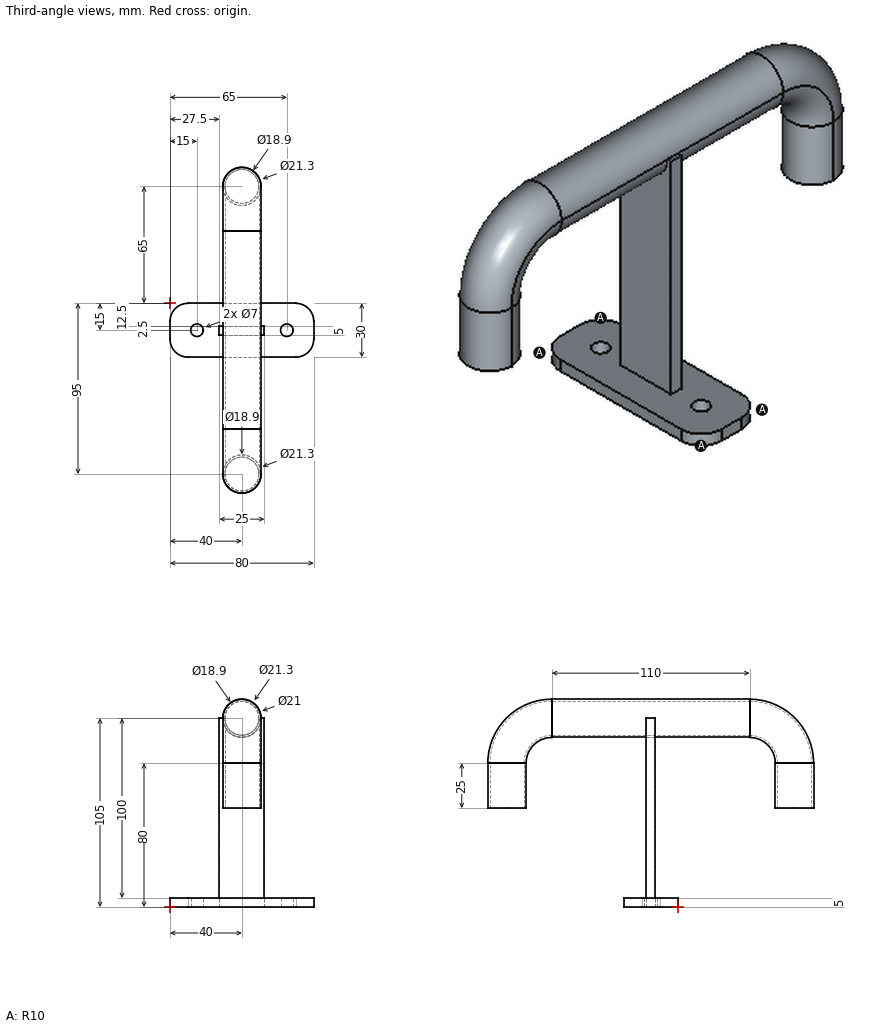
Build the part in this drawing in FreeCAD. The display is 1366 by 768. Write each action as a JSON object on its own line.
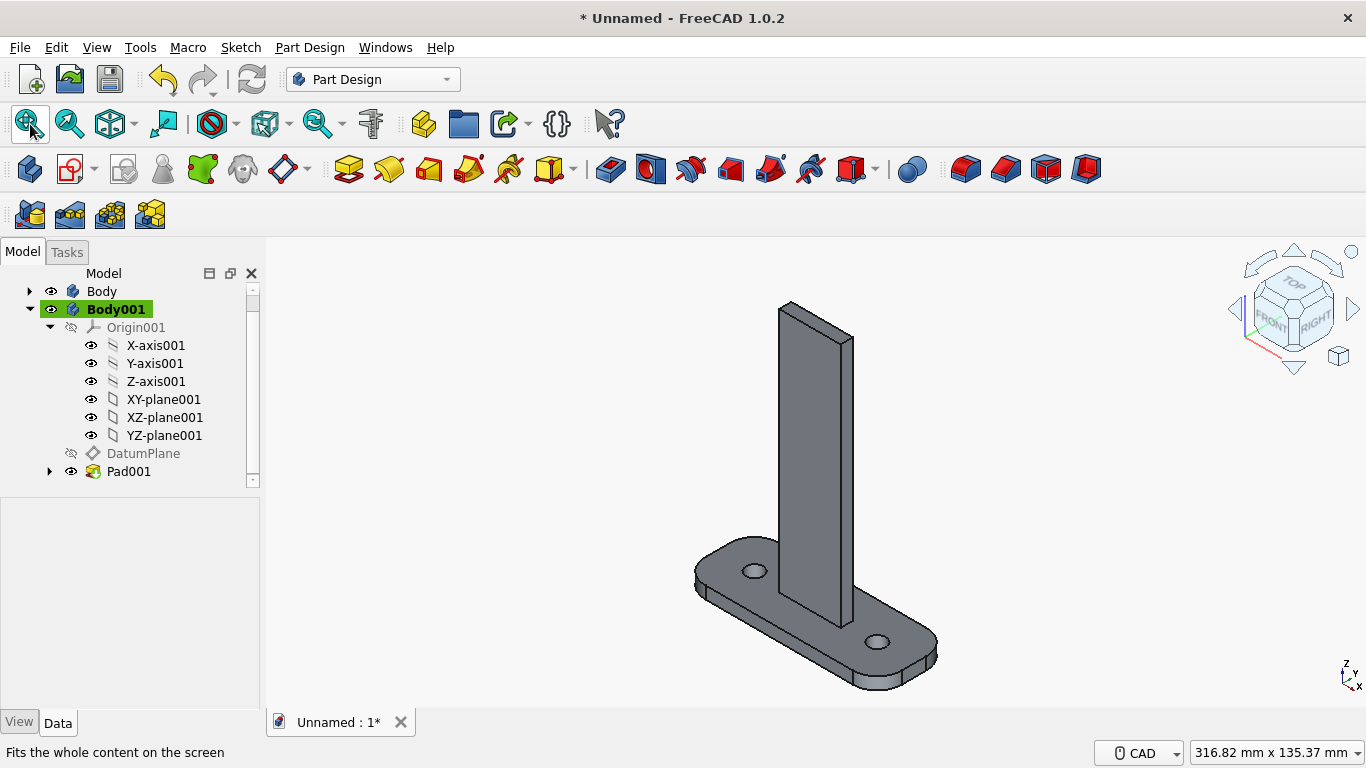
{"action": "left_click", "coordinate": [810, 386]}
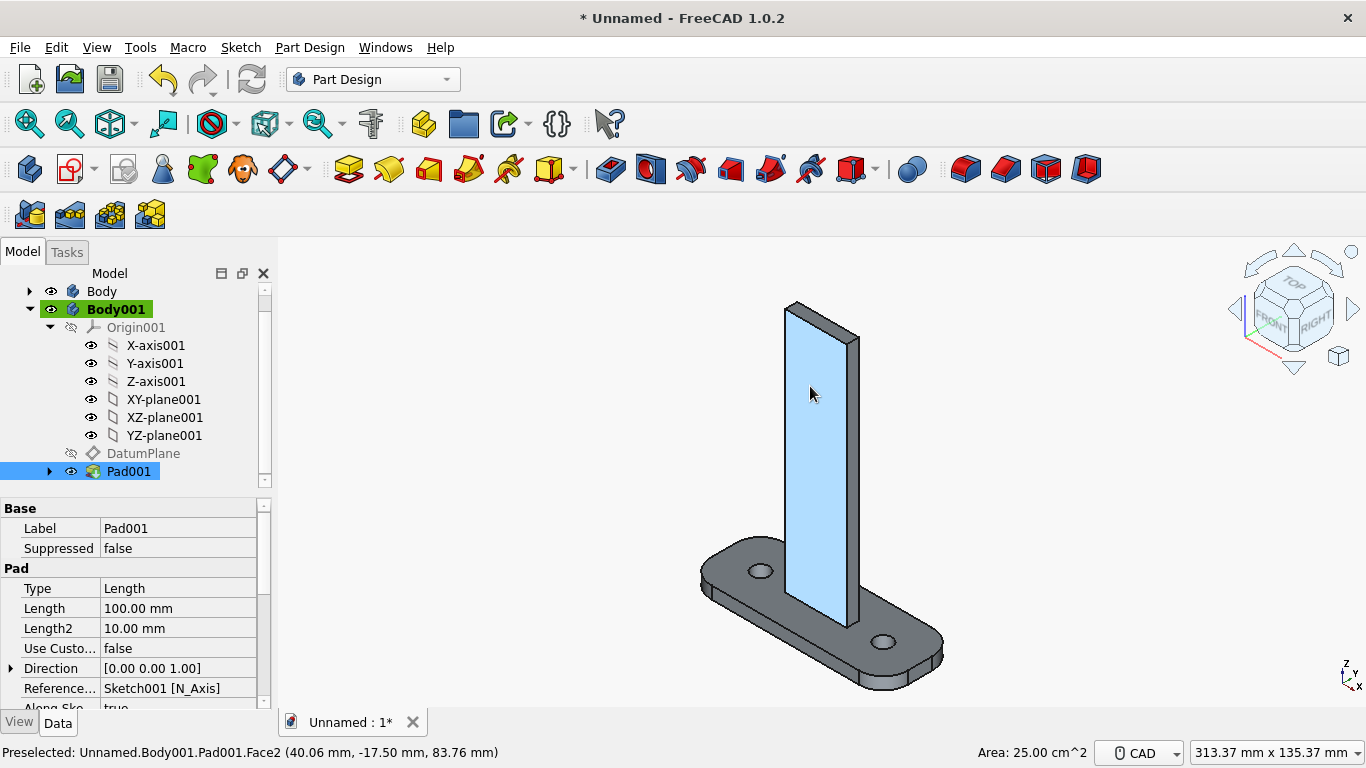
{"action": "left_click", "coordinate": [70, 170]}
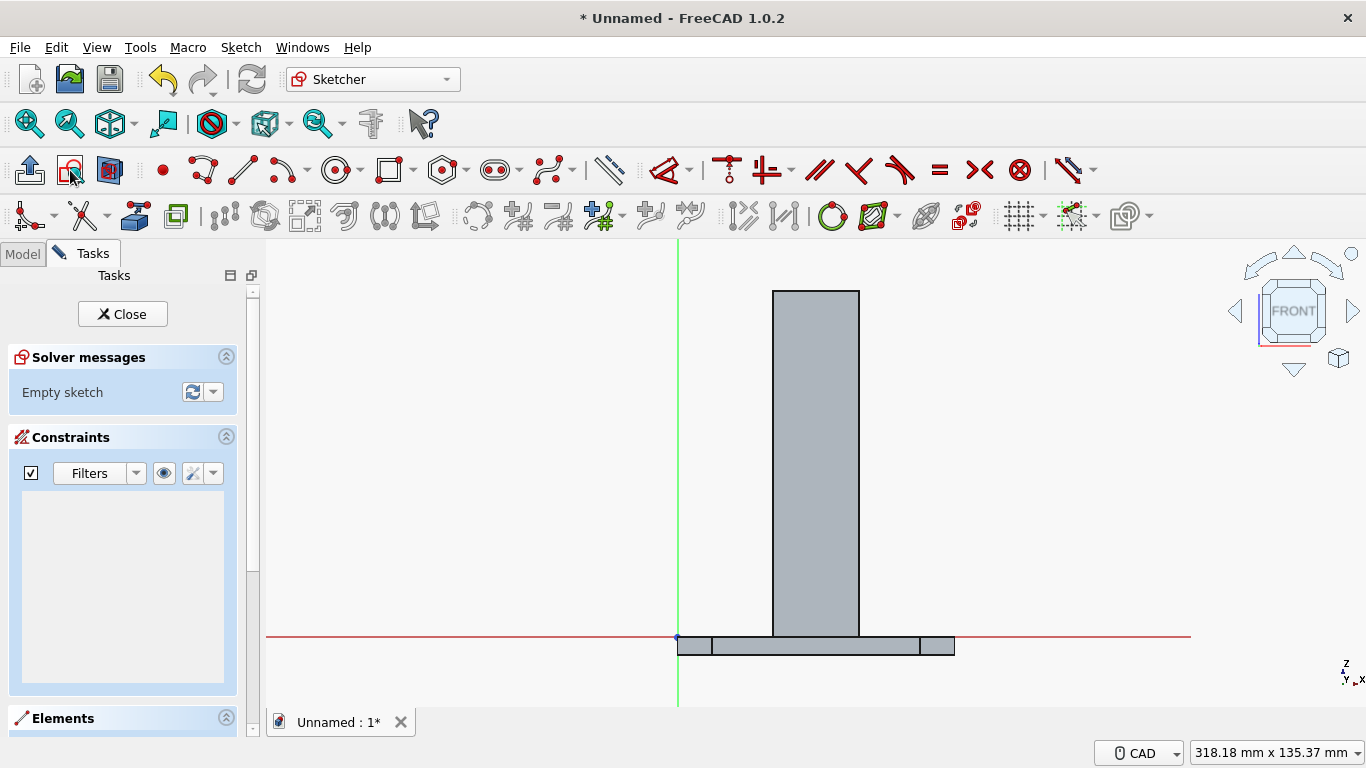
{"action": "scroll", "coordinate": [748, 473], "scroll_direction": "down", "scroll_amount": 5}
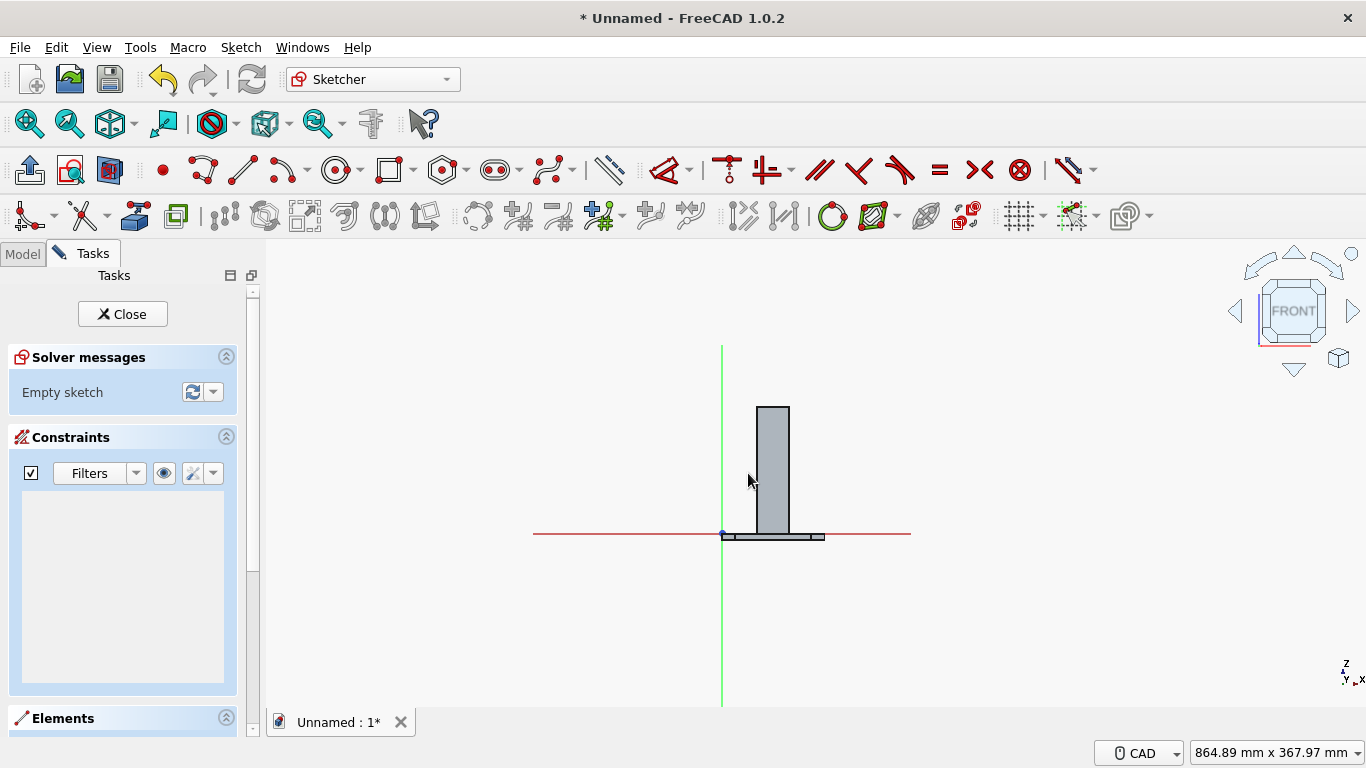
{"action": "scroll", "coordinate": [776, 400], "scroll_direction": "up", "scroll_amount": 12}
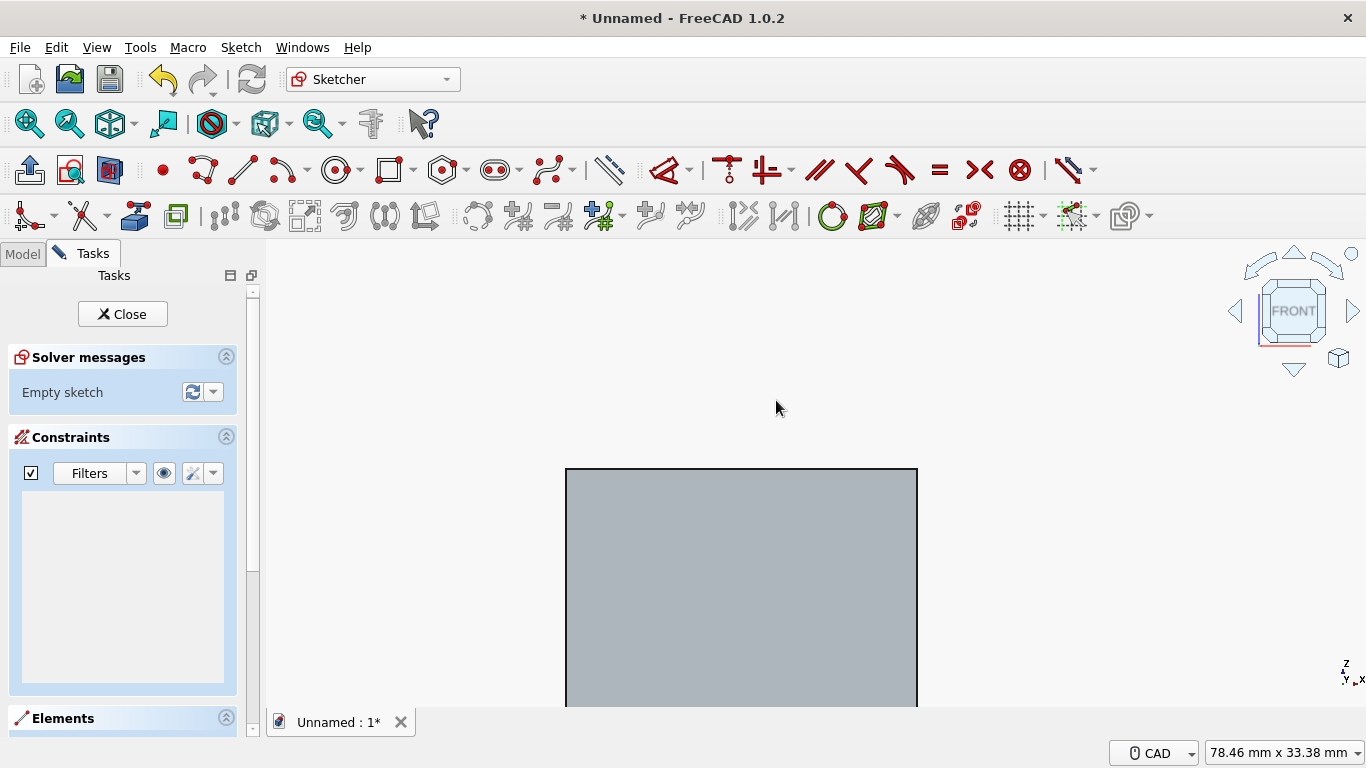
{"action": "left_click", "coordinate": [336, 170]}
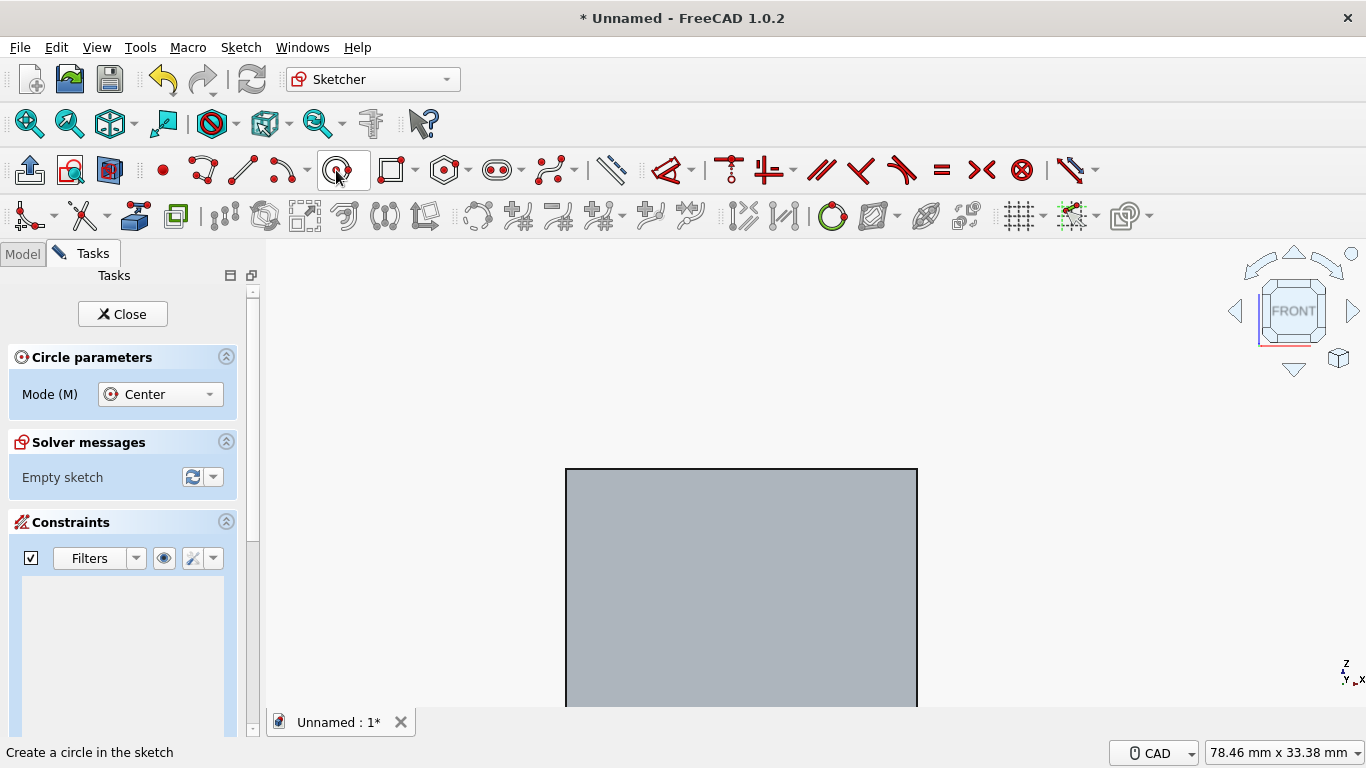
{"action": "left_click", "coordinate": [742, 469]}
{"action": "mouse_move", "coordinate": [846, 365]}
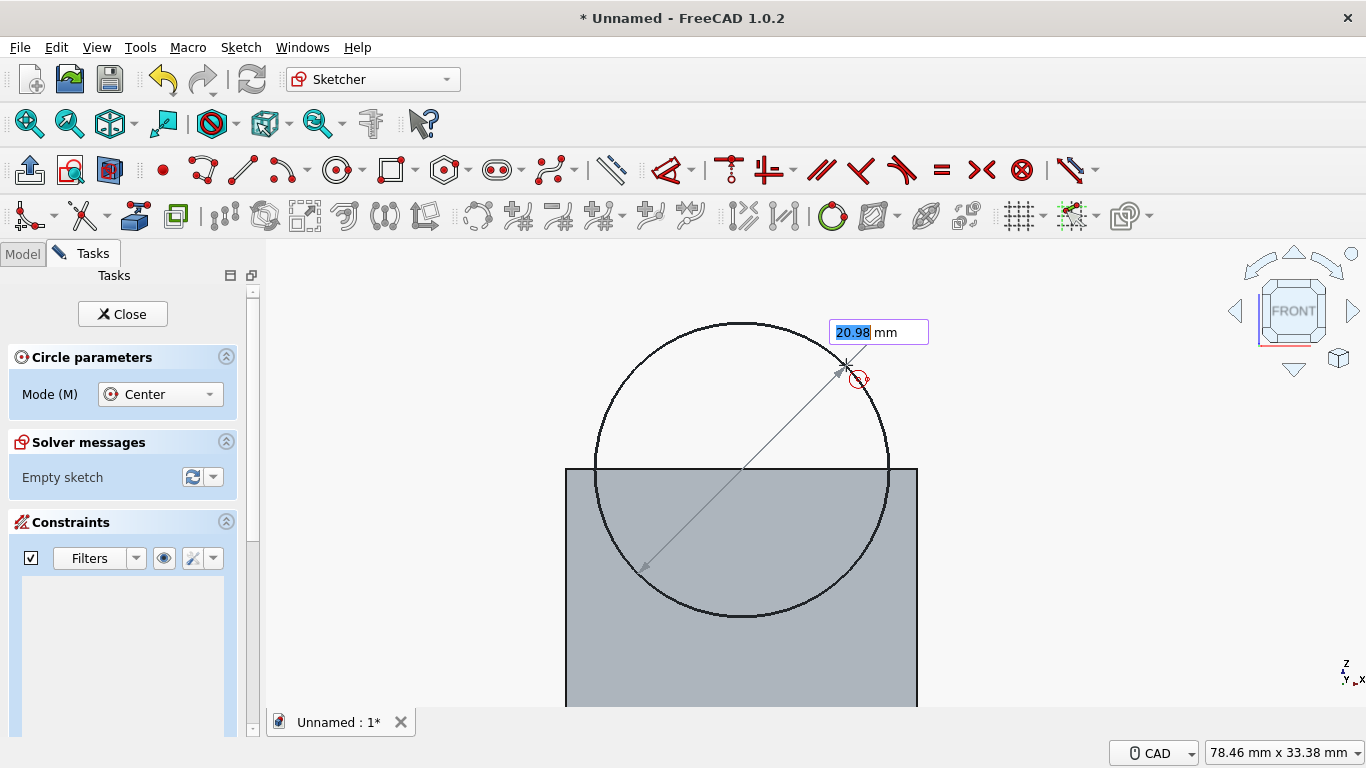
{"action": "type", "text": "21"}
{"action": "key", "text": "Return"}
{"action": "key", "text": "Escape"}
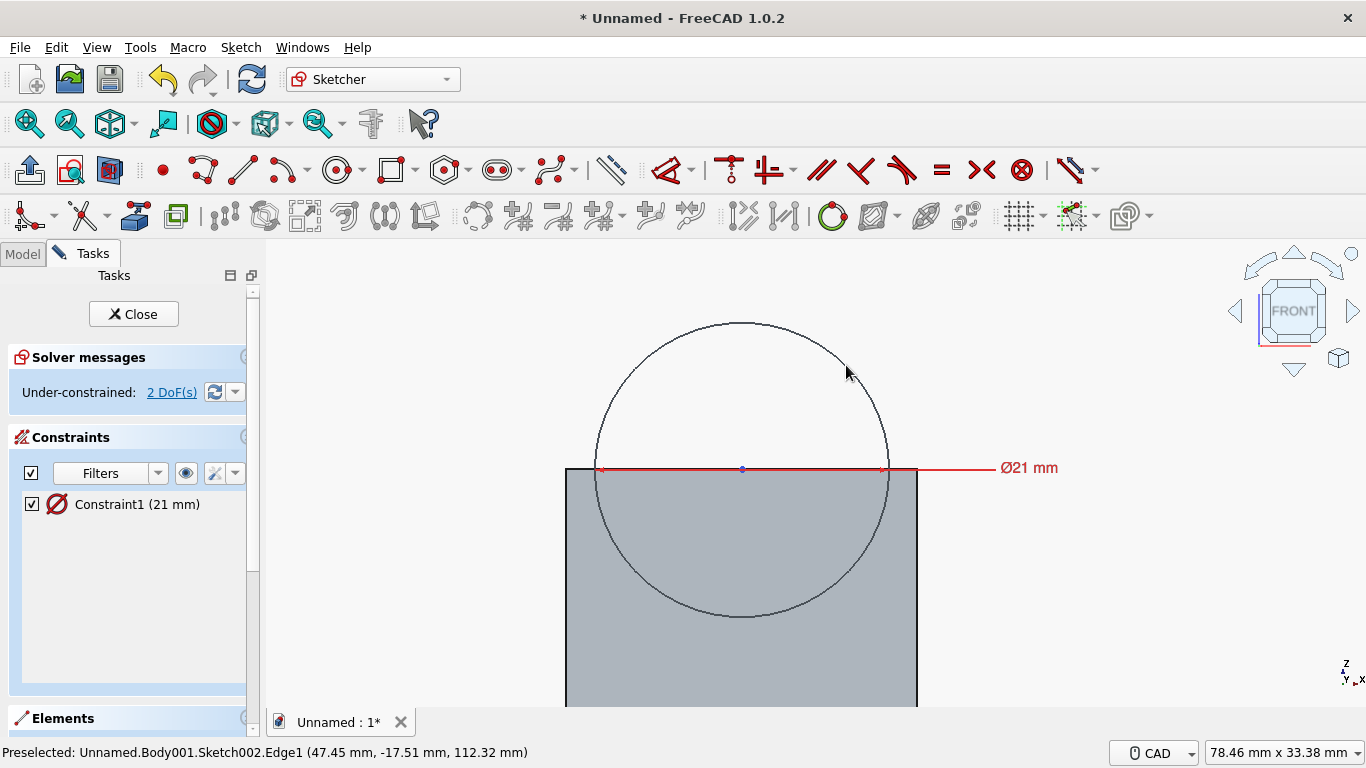
{"action": "left_click", "coordinate": [666, 170]}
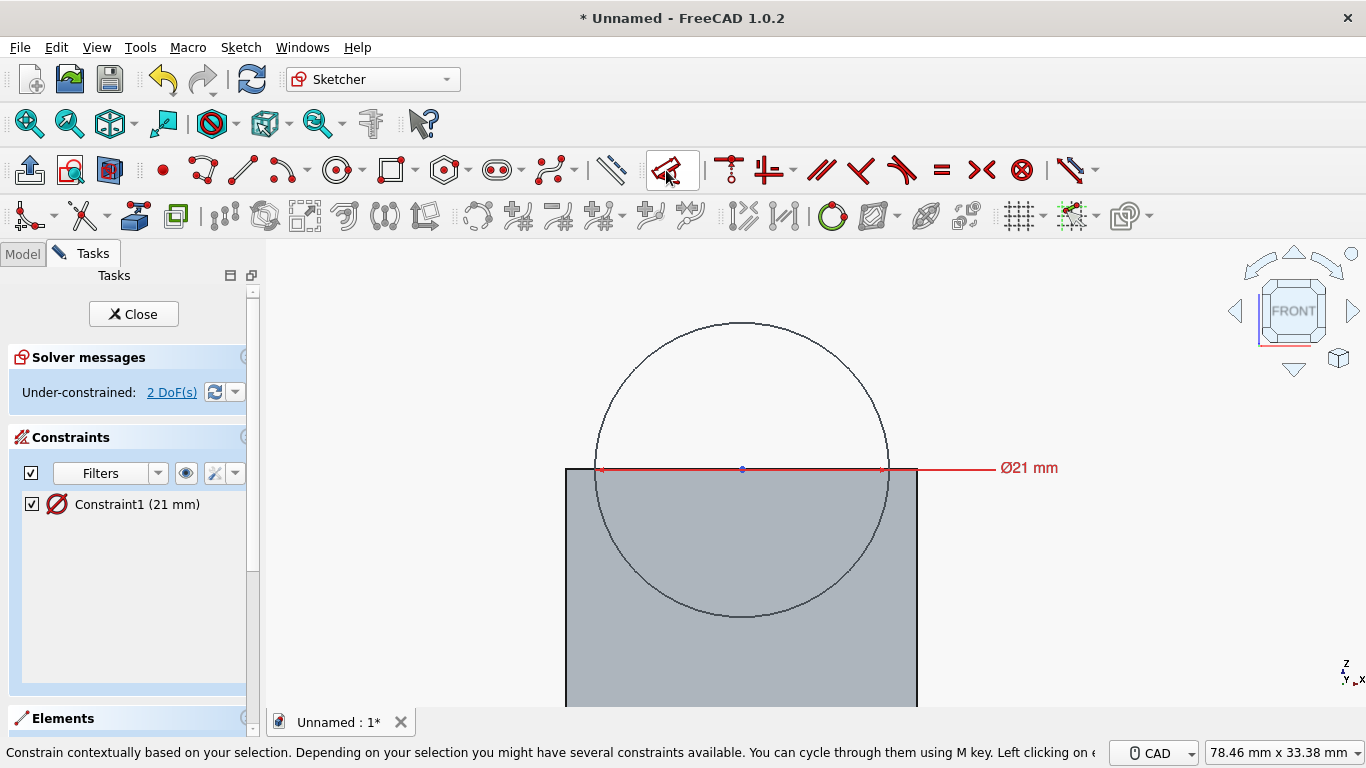
{"action": "left_click", "coordinate": [742, 470]}
{"action": "left_click", "coordinate": [518, 436]}